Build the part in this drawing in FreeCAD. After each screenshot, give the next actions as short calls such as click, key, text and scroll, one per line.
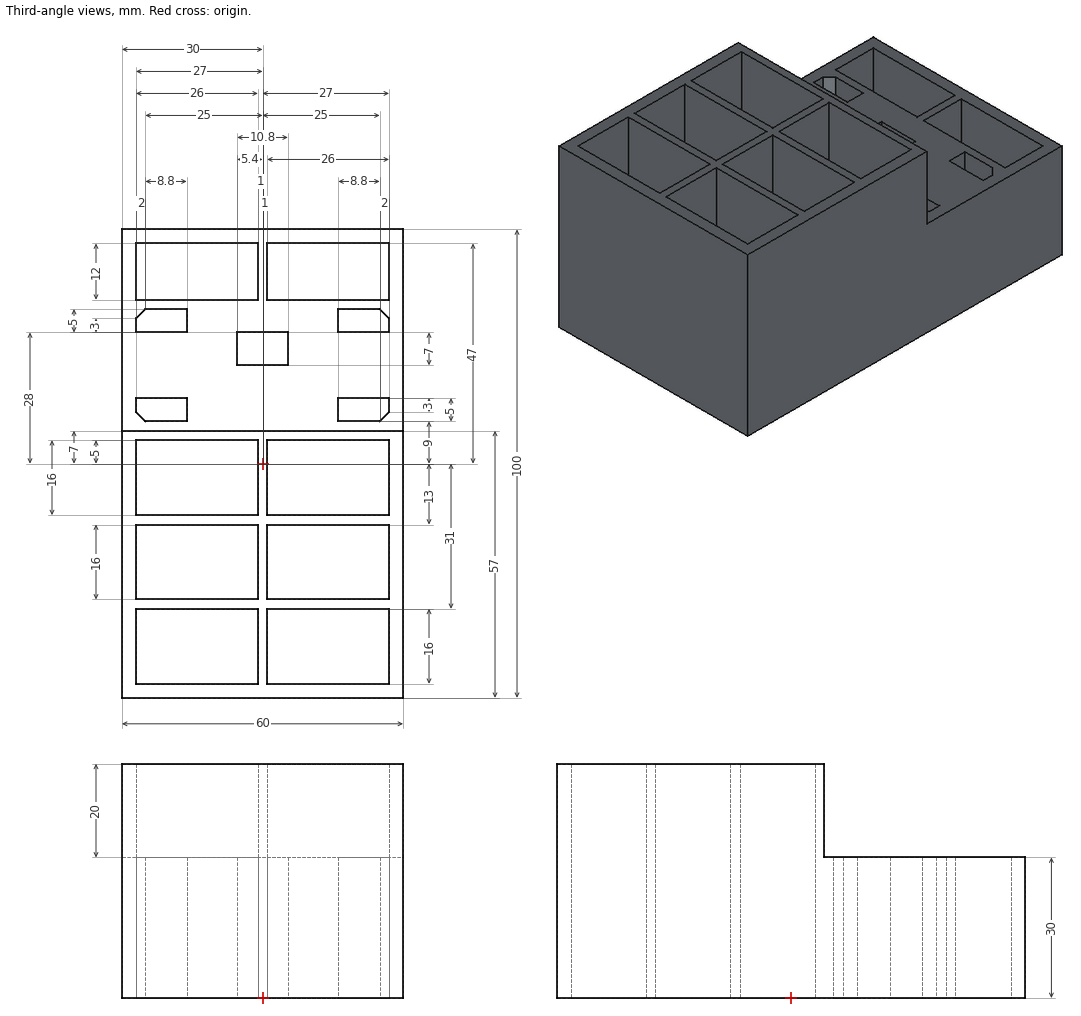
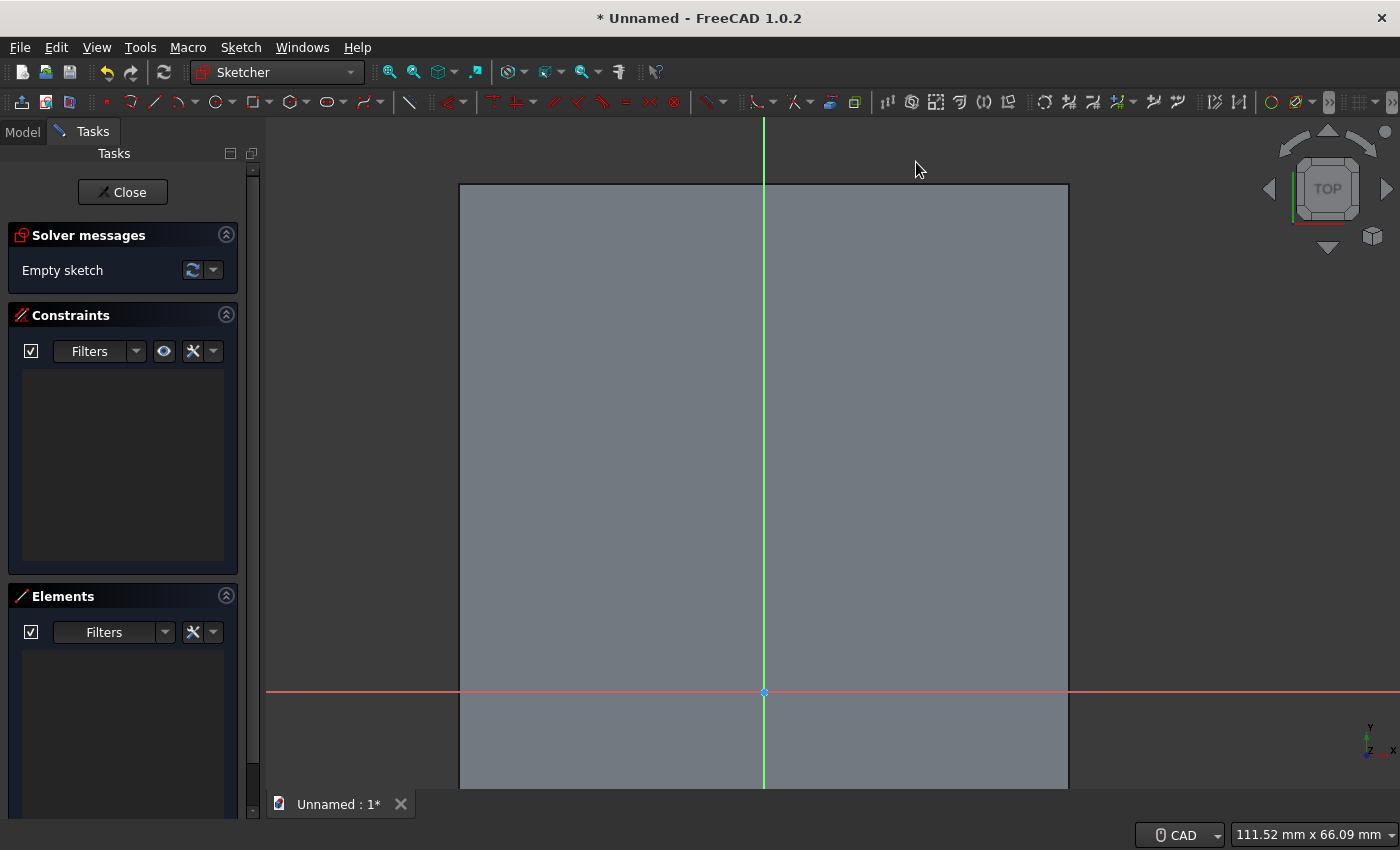
click(254, 102)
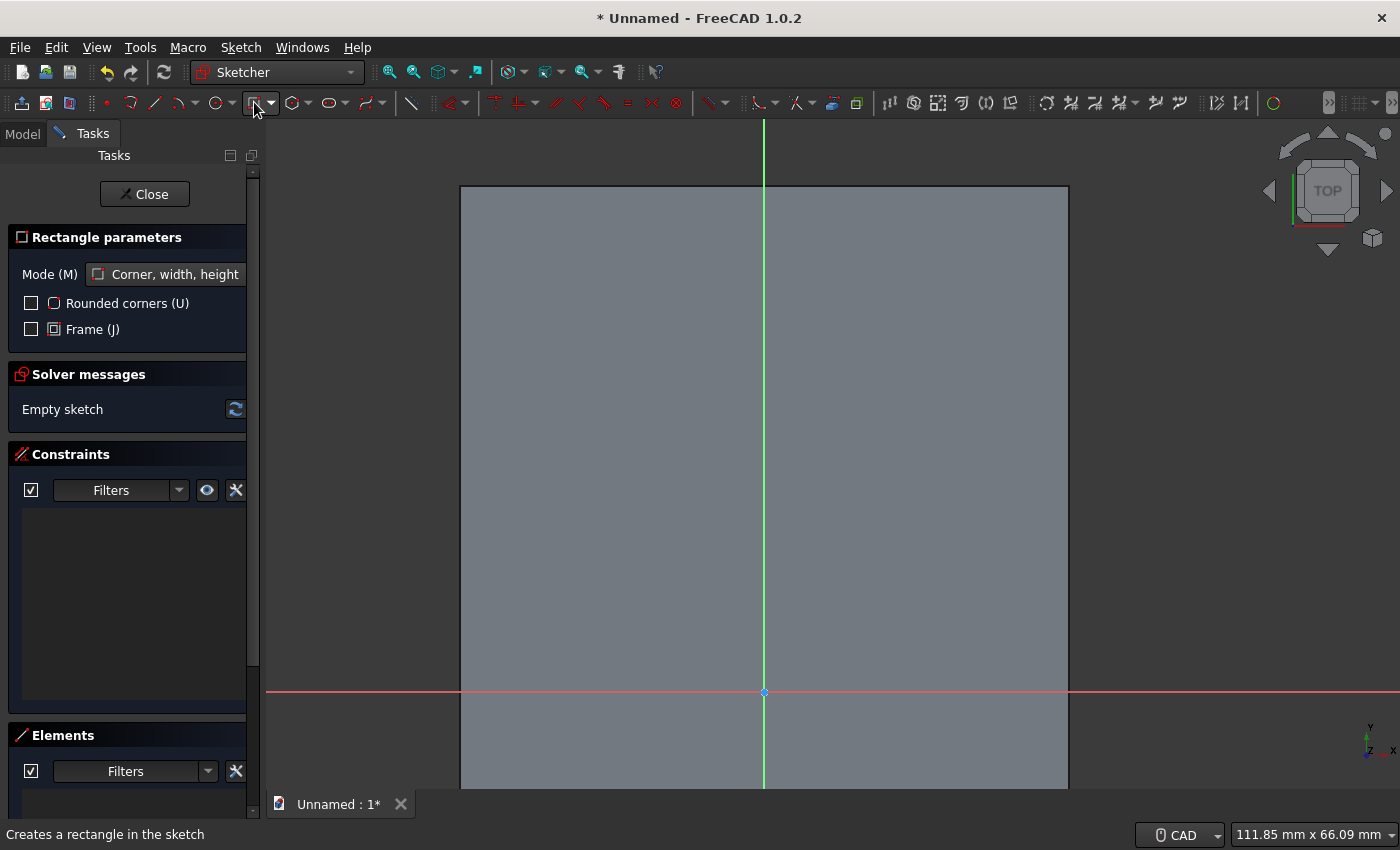
scroll(775, 216, up, 3)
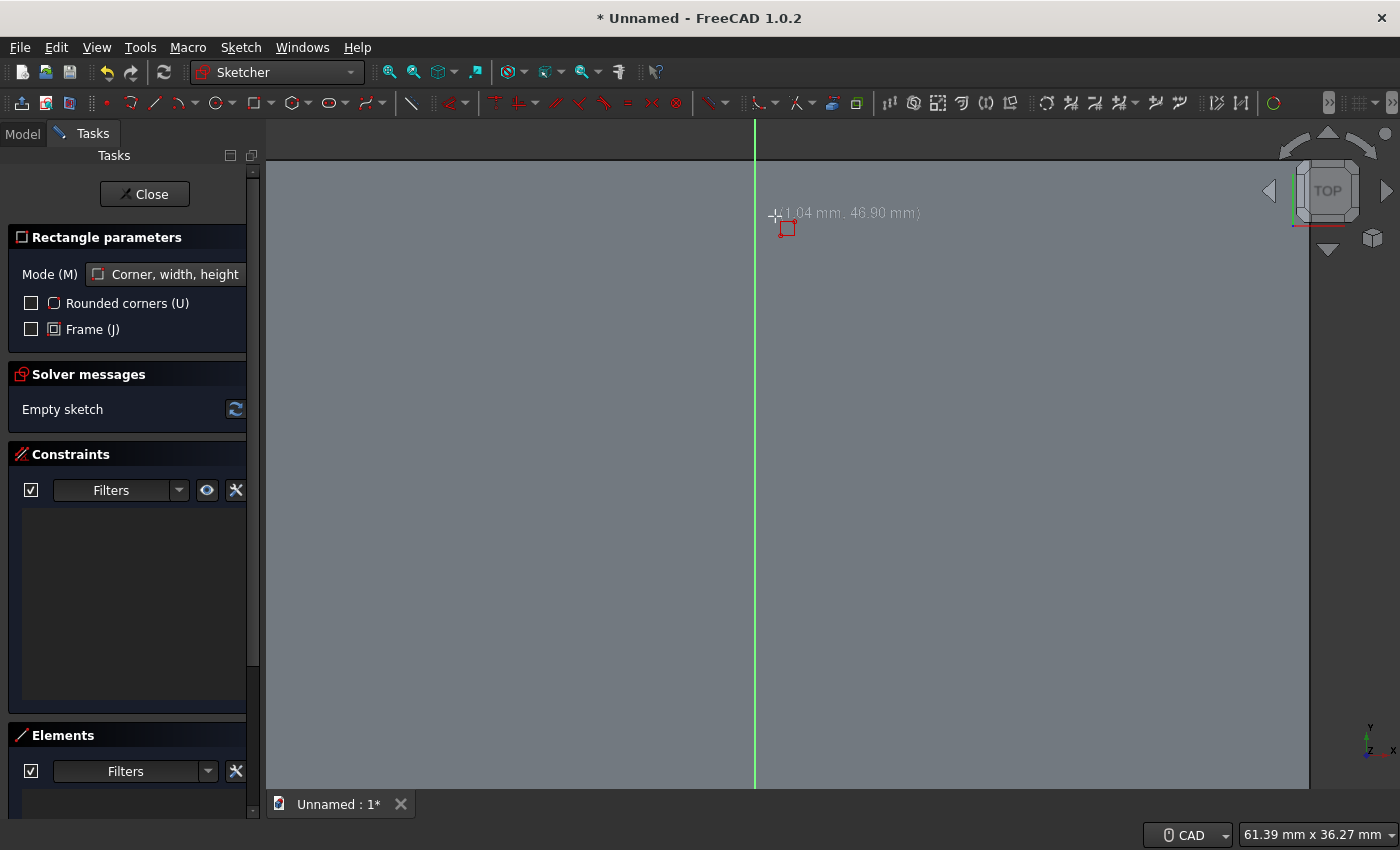
click(774, 216)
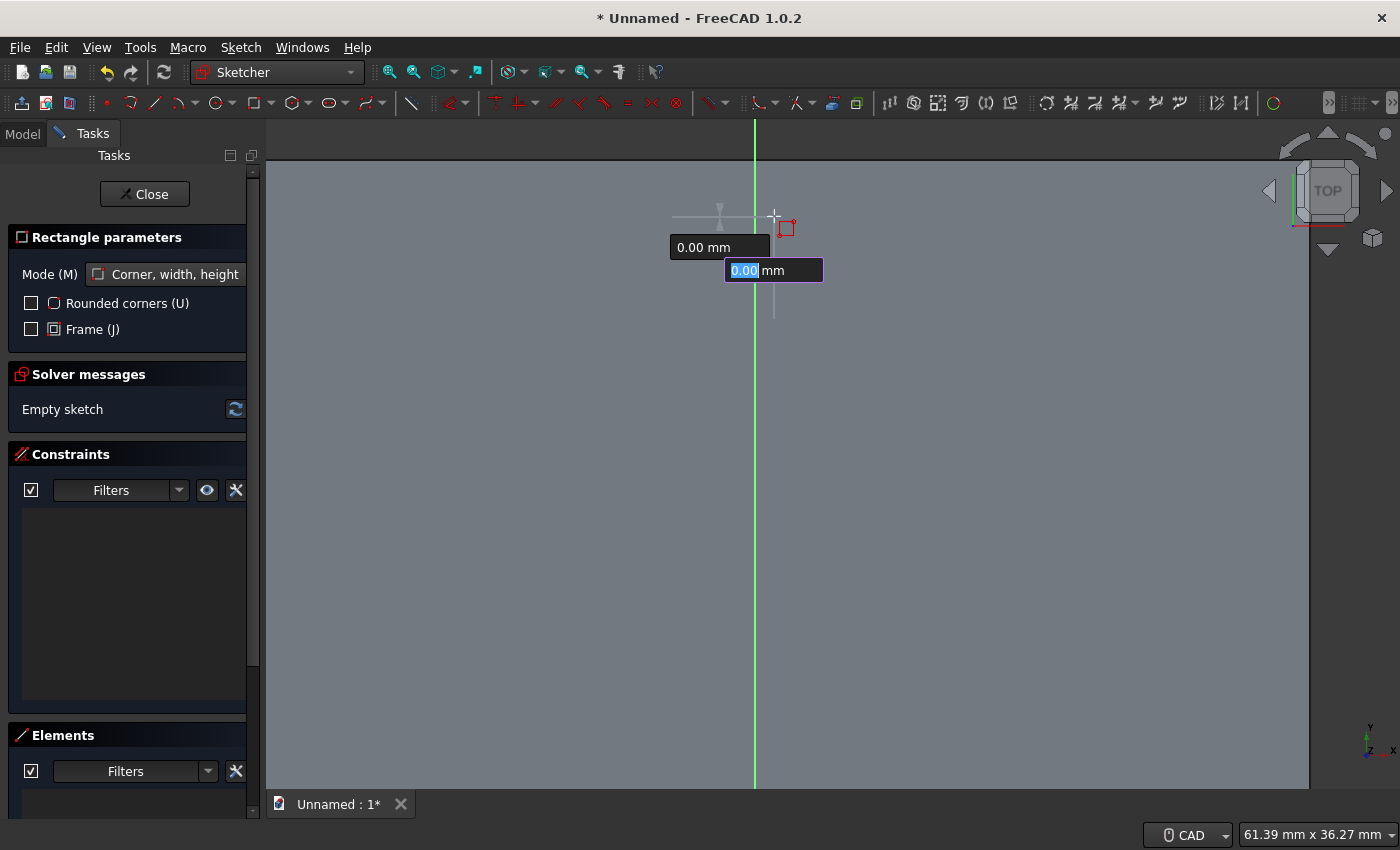
scroll(775, 216, down, 3)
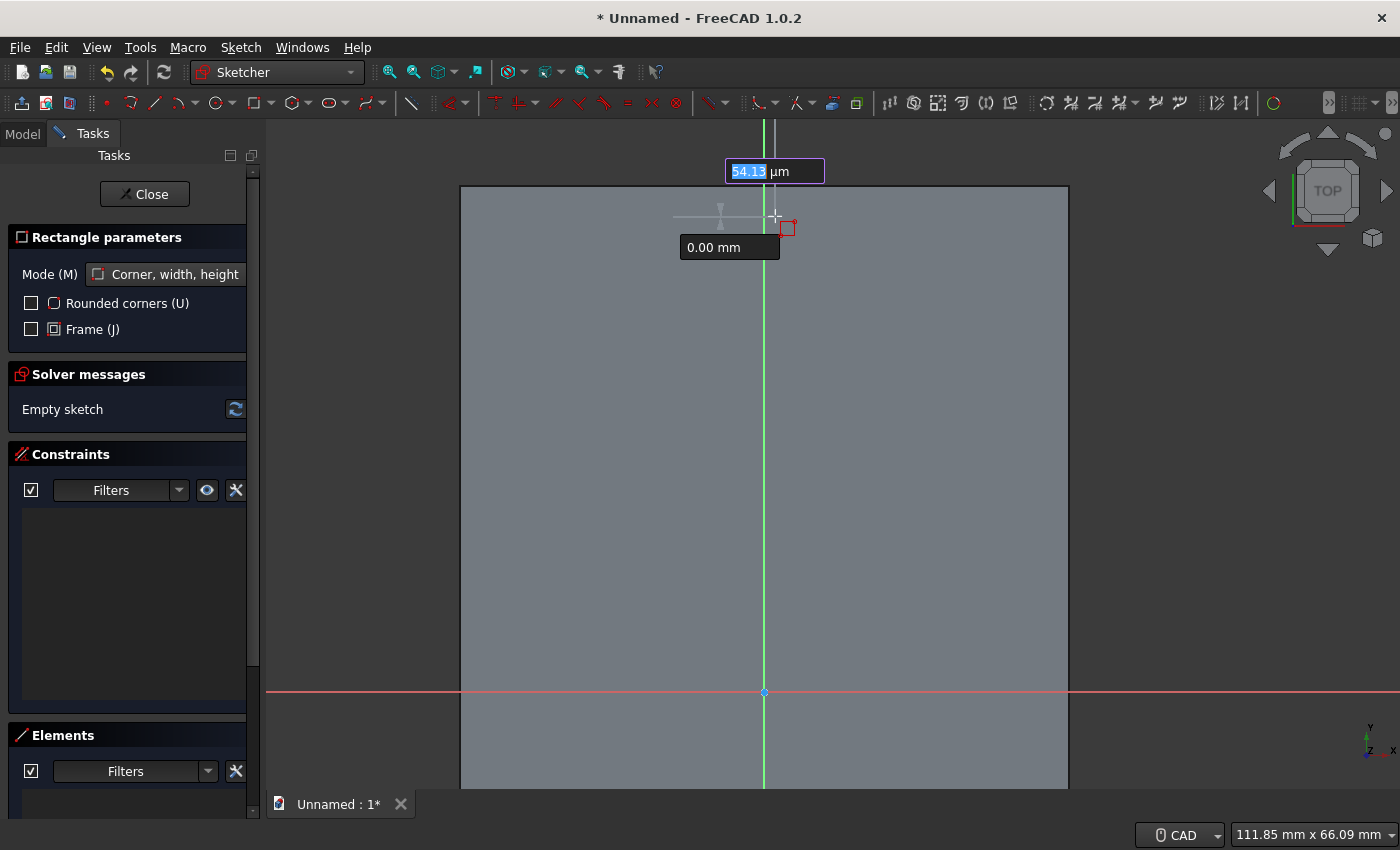
click(1038, 338)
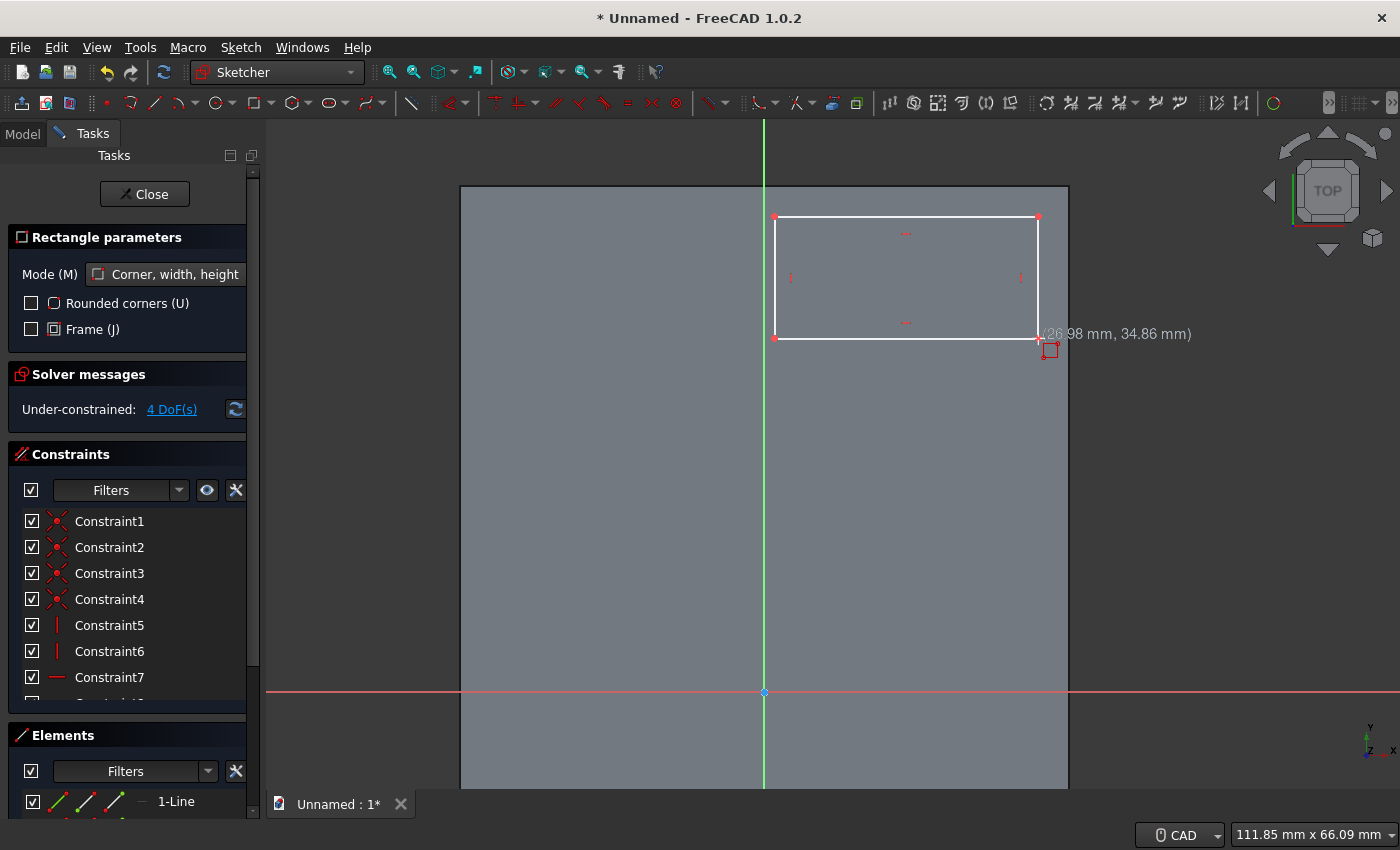
click(491, 216)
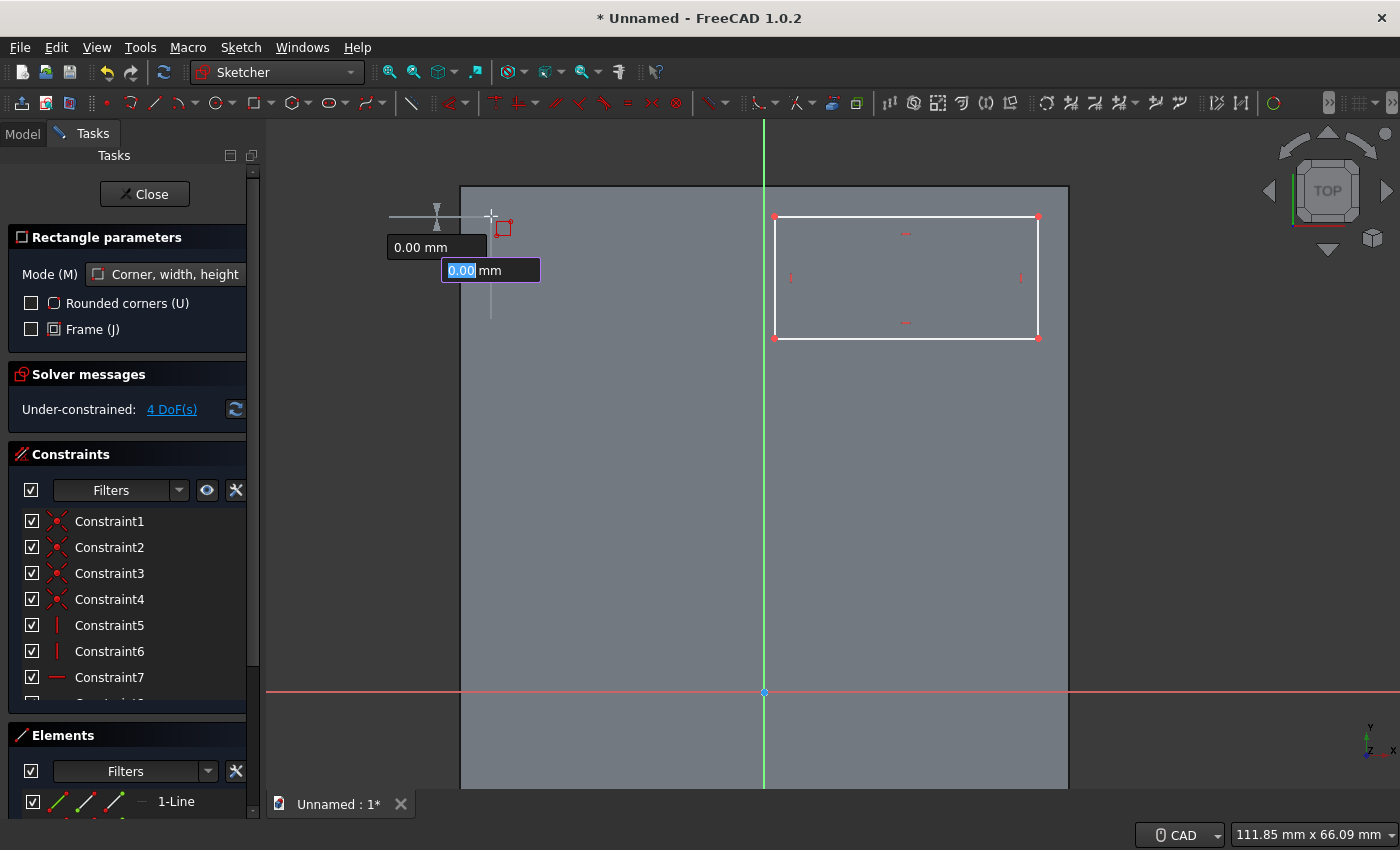
scroll(754, 338, up, 3)
move(754, 337)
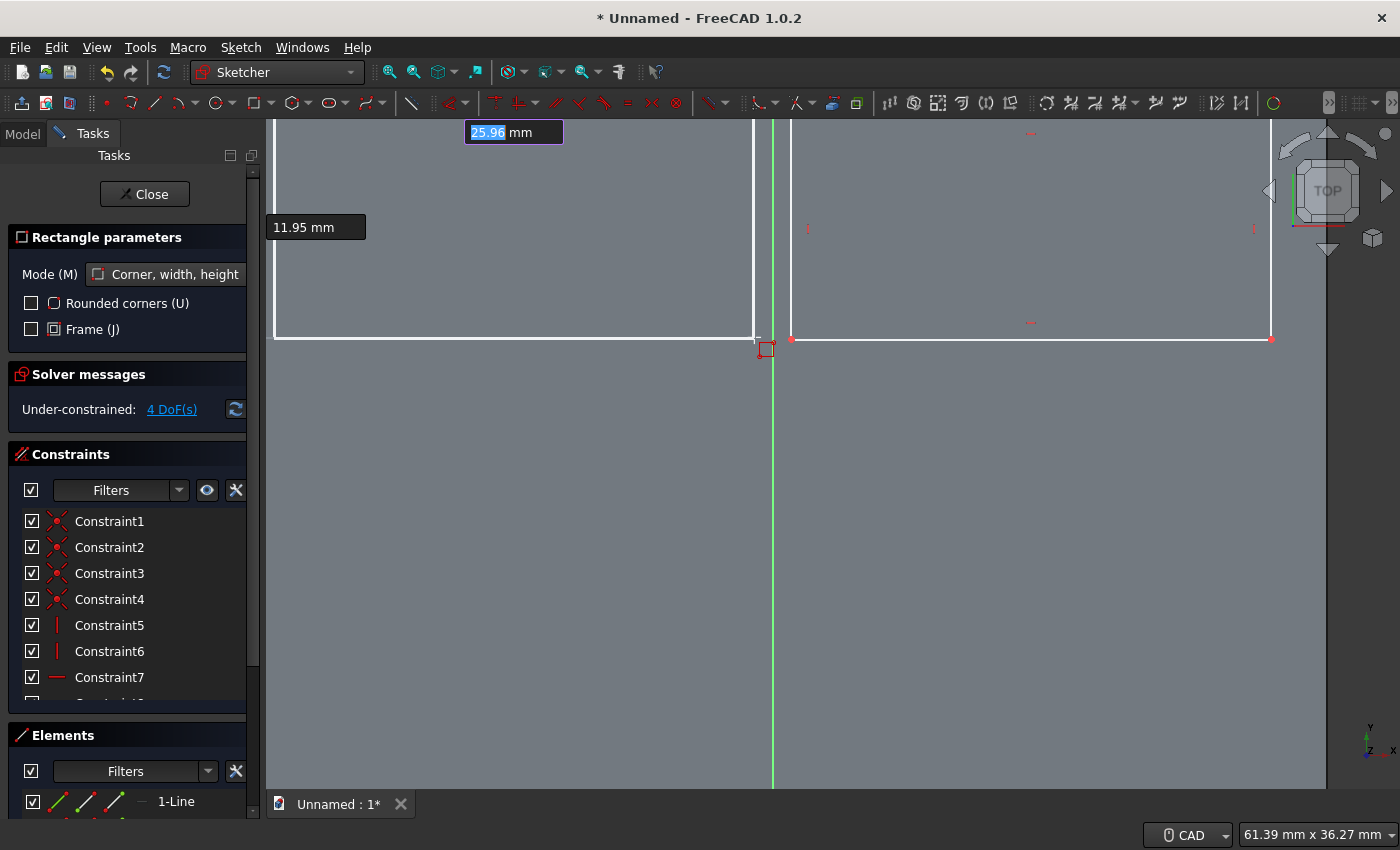
text(26)
key(Tab)
text(12)
key(Return)
key(Escape)